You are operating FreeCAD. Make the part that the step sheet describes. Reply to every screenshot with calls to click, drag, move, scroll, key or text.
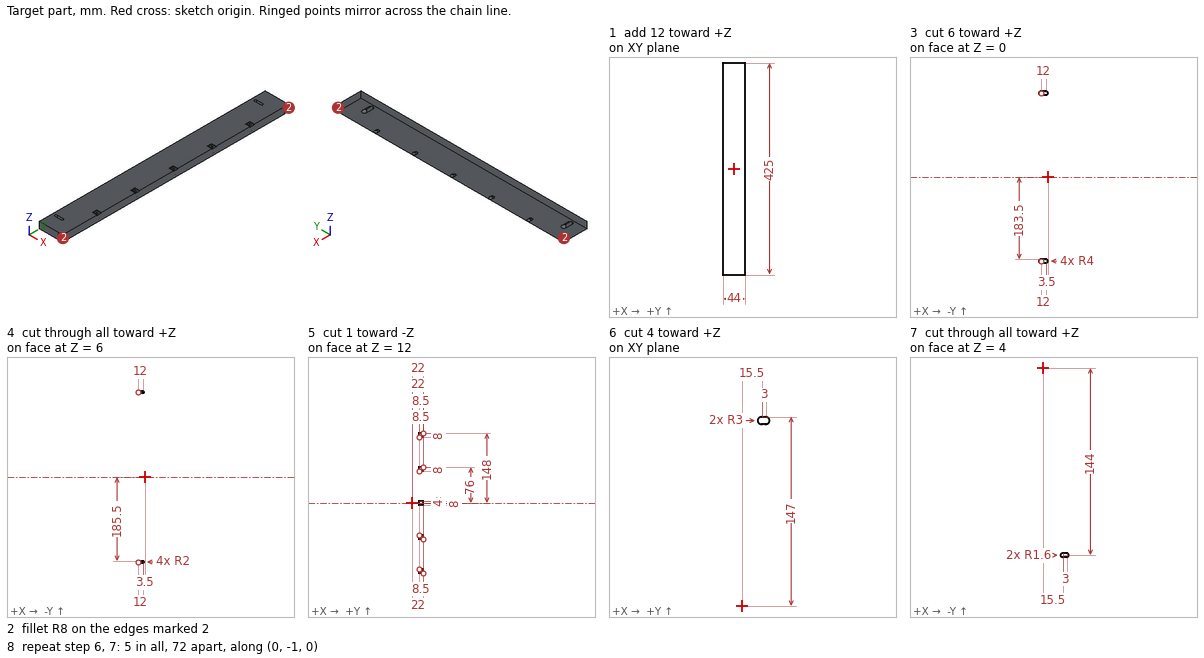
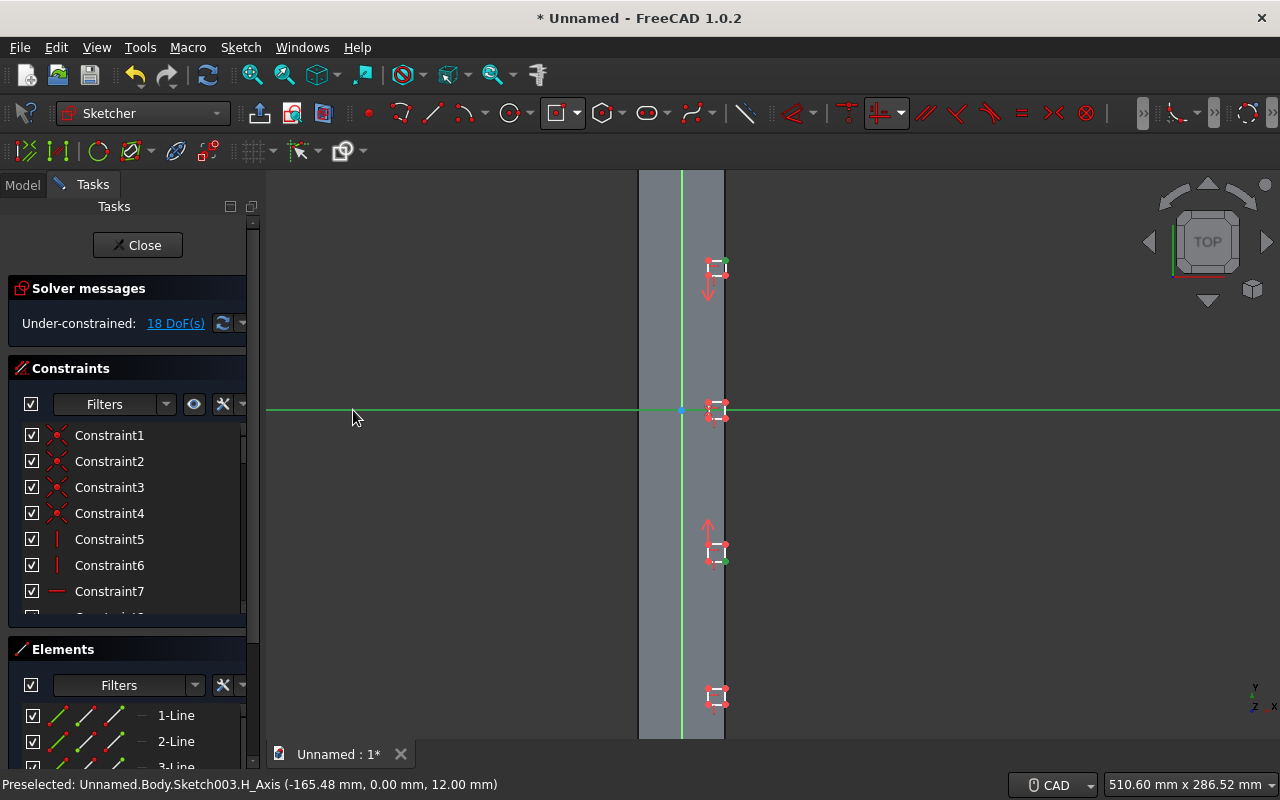
key(s)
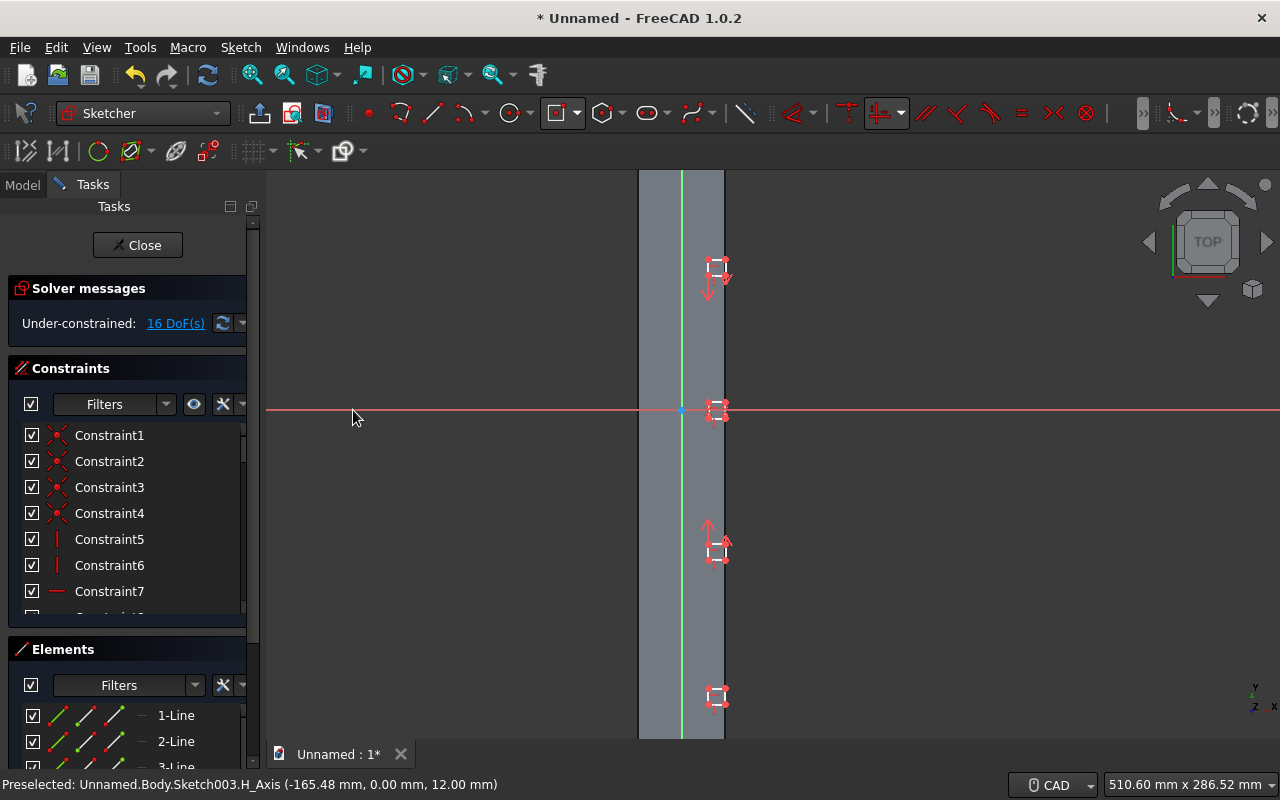
scroll(707, 545, down, 2)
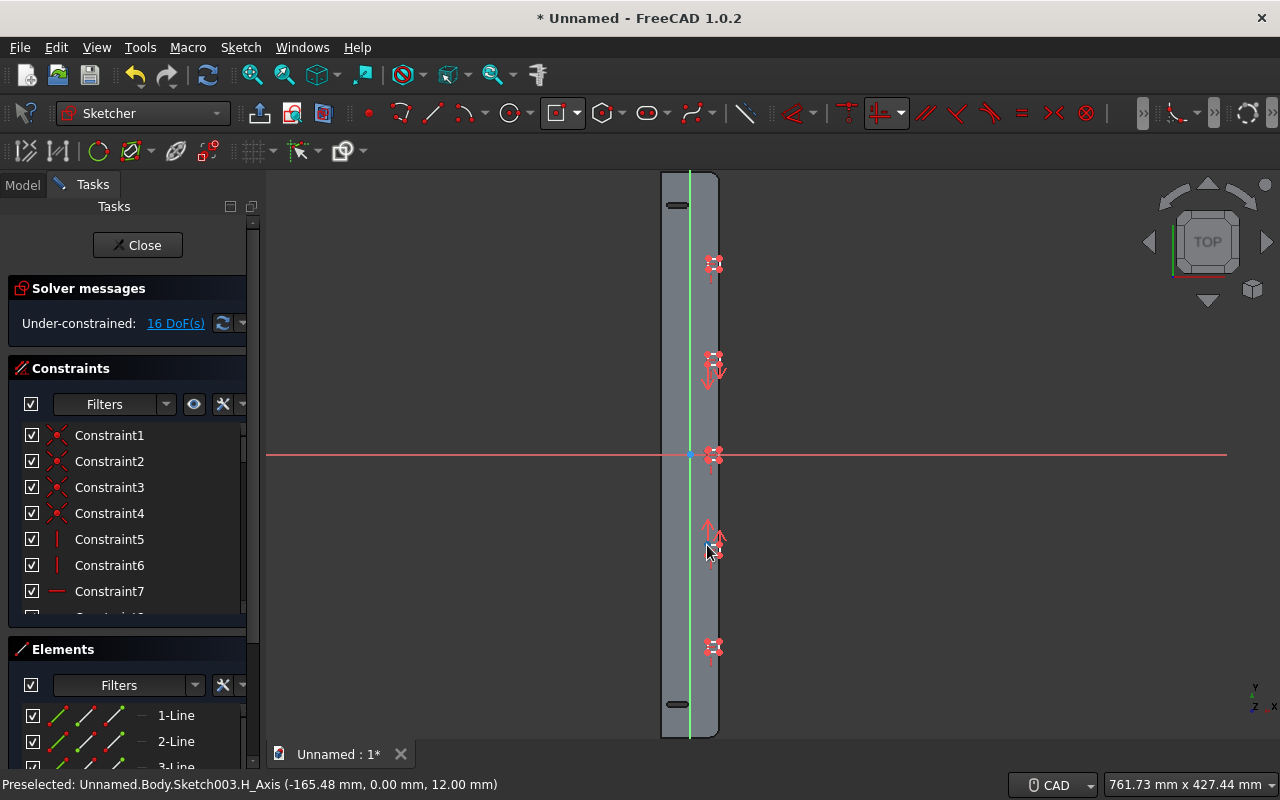
click(708, 269)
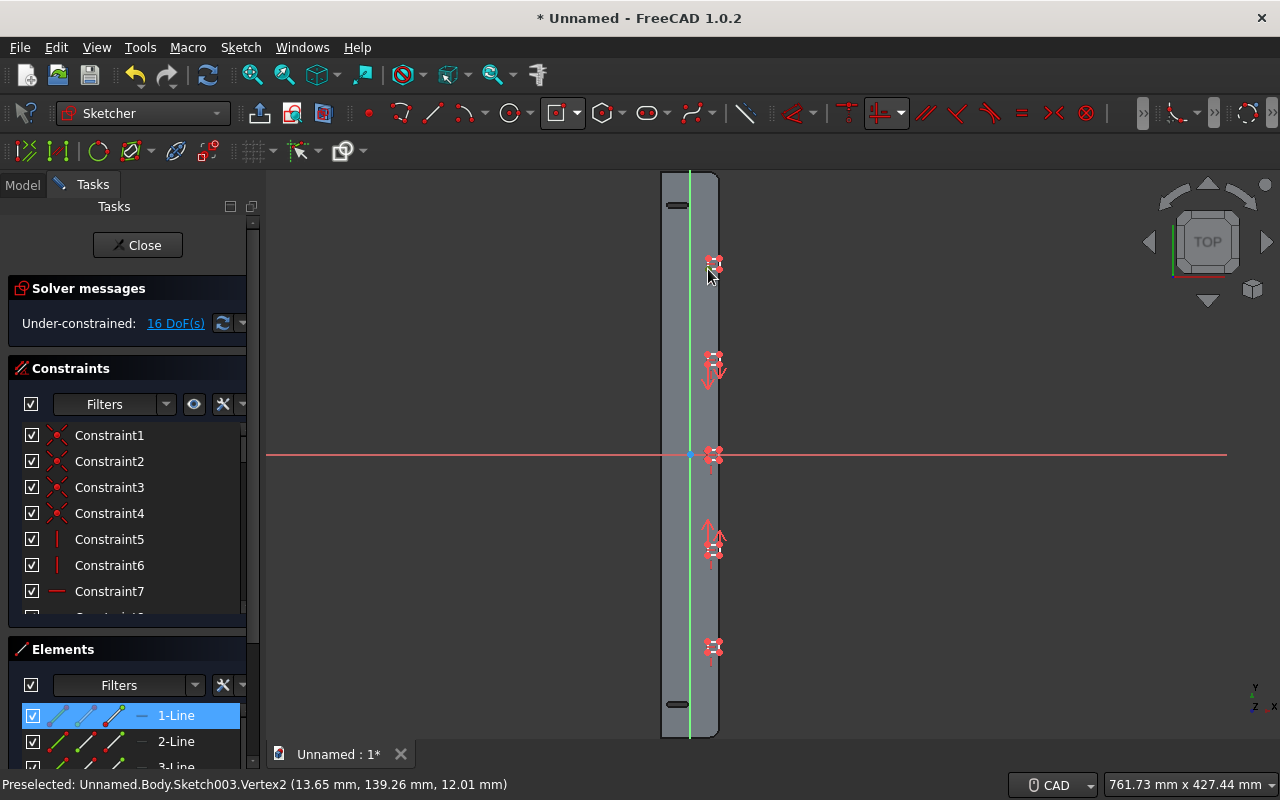
click(708, 642)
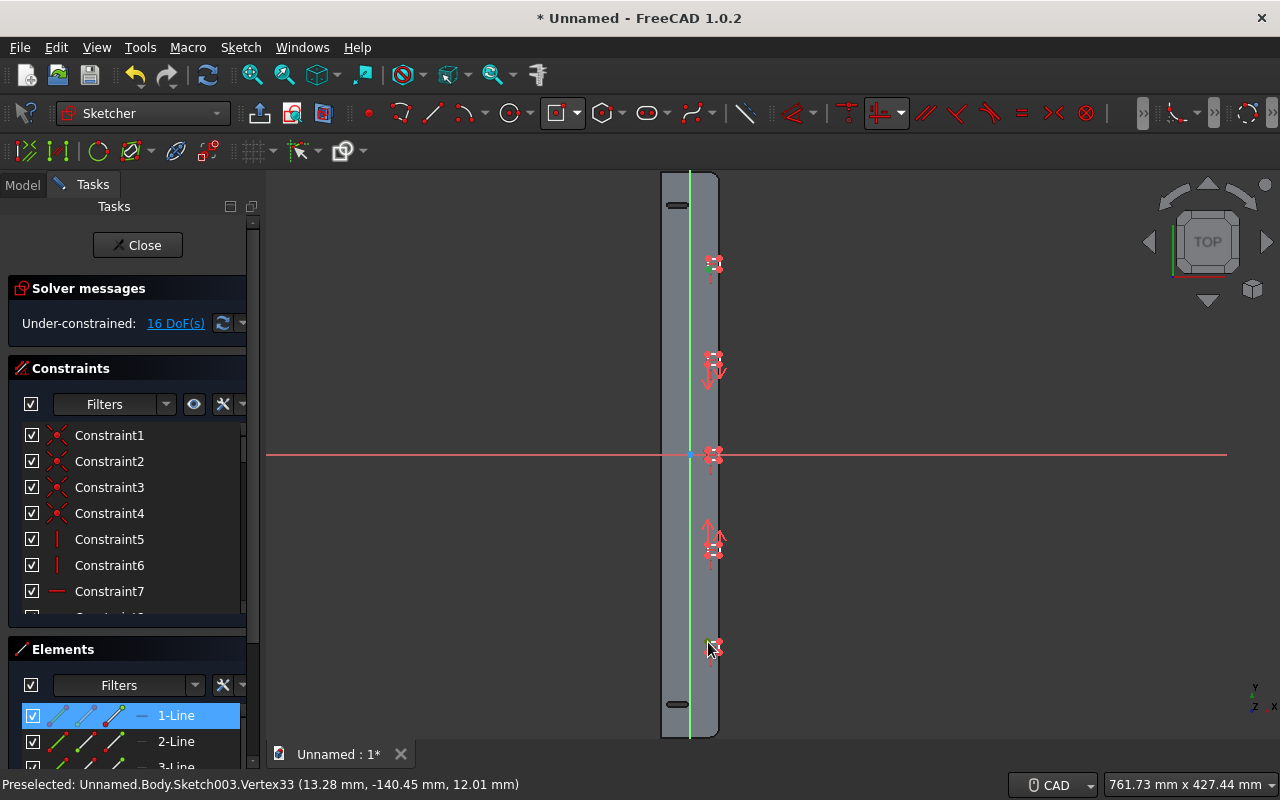
click(353, 455)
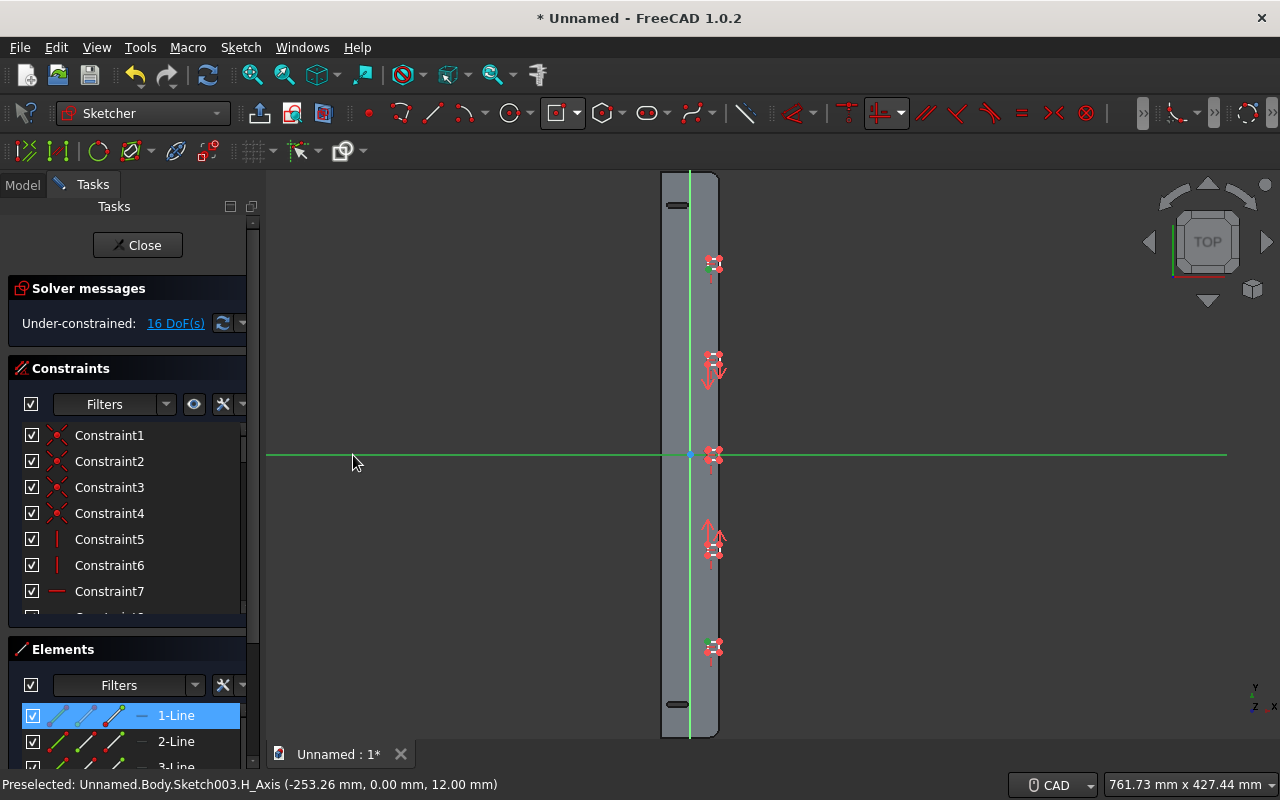
click(1054, 114)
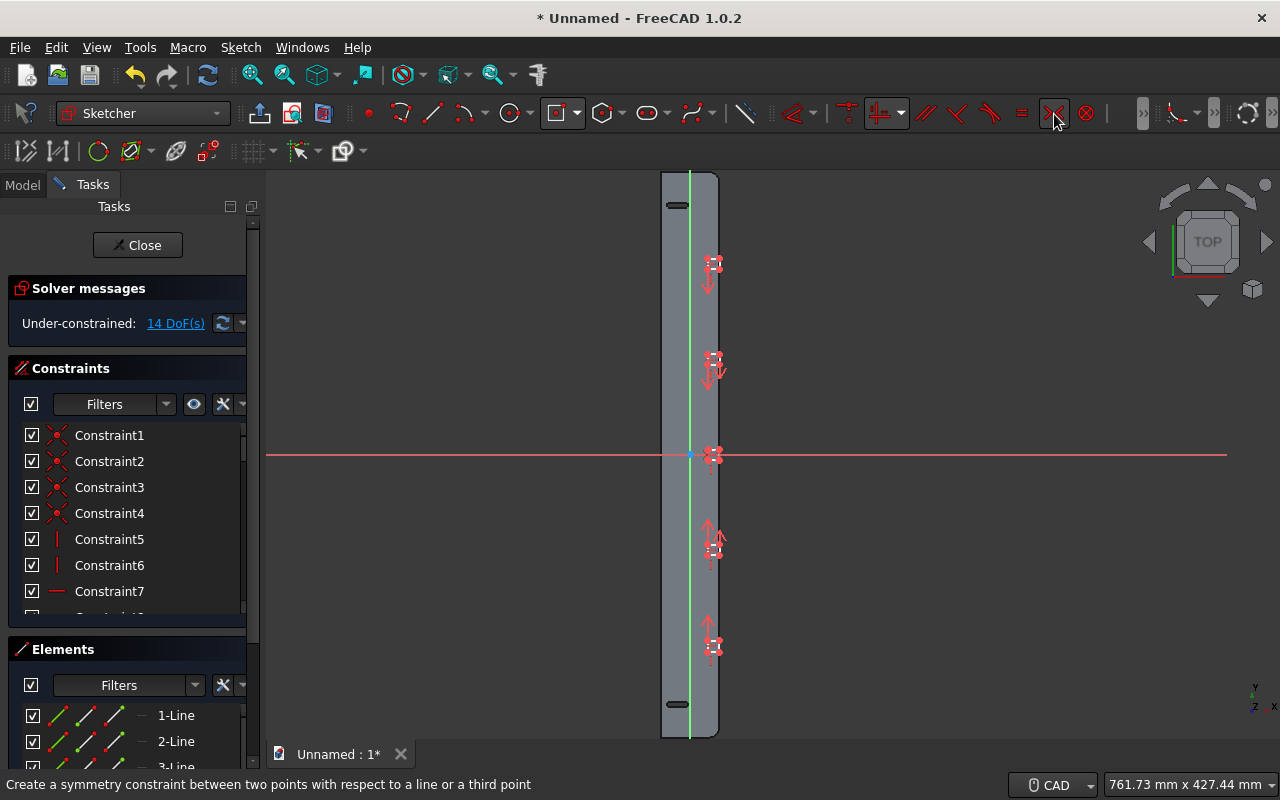
click(720, 259)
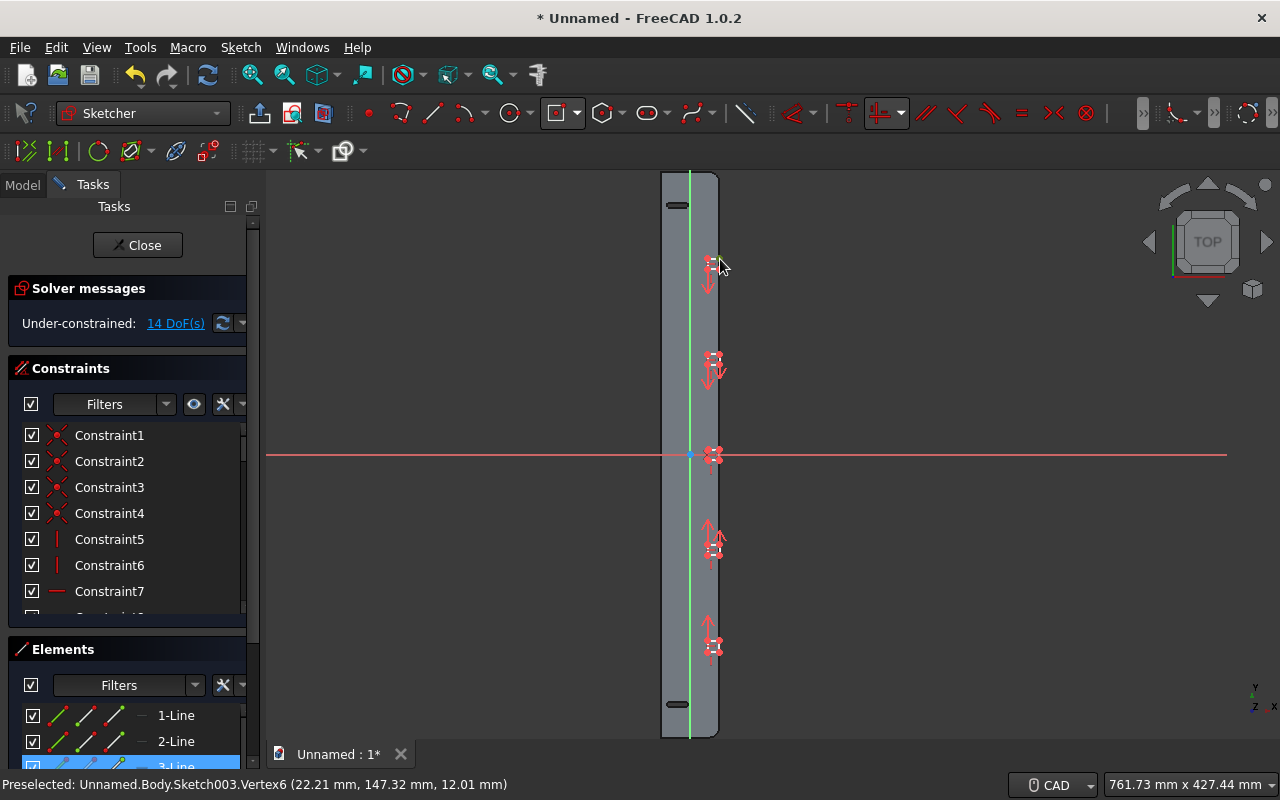
click(719, 652)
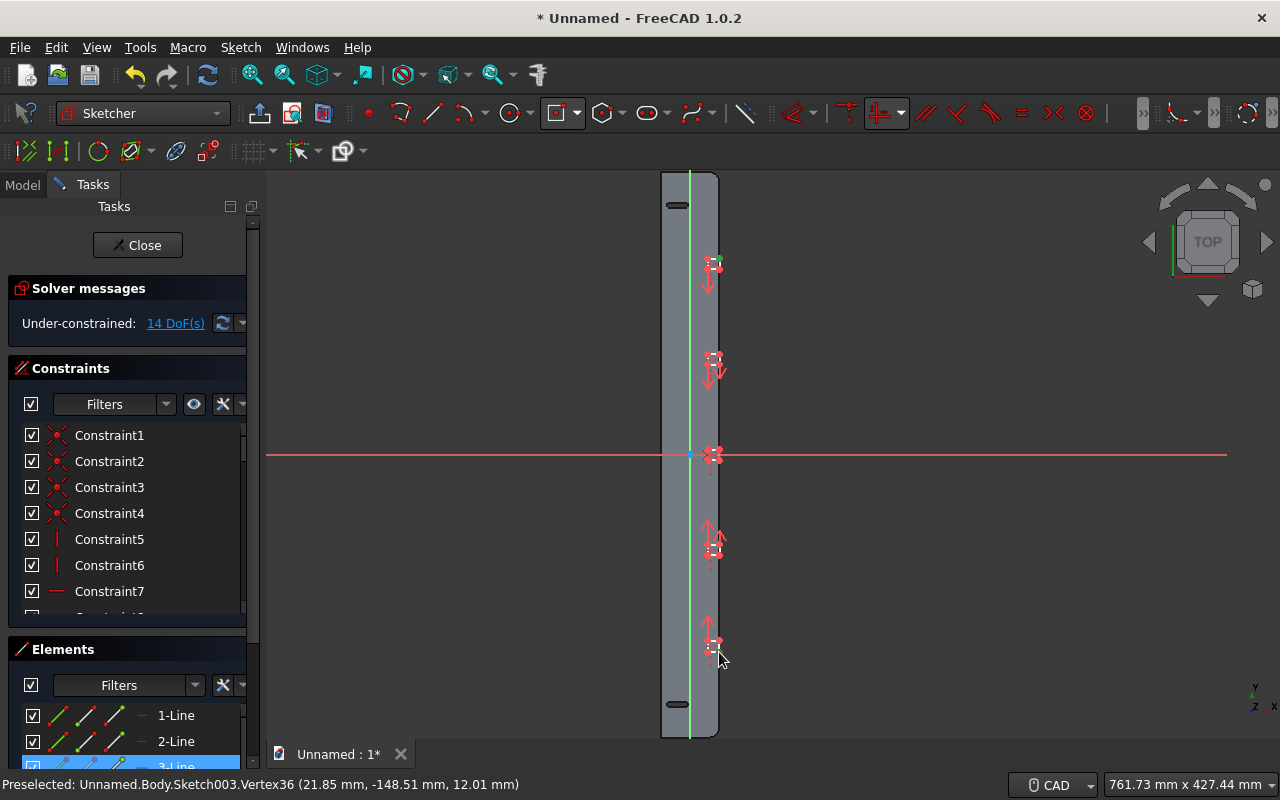
click(353, 455)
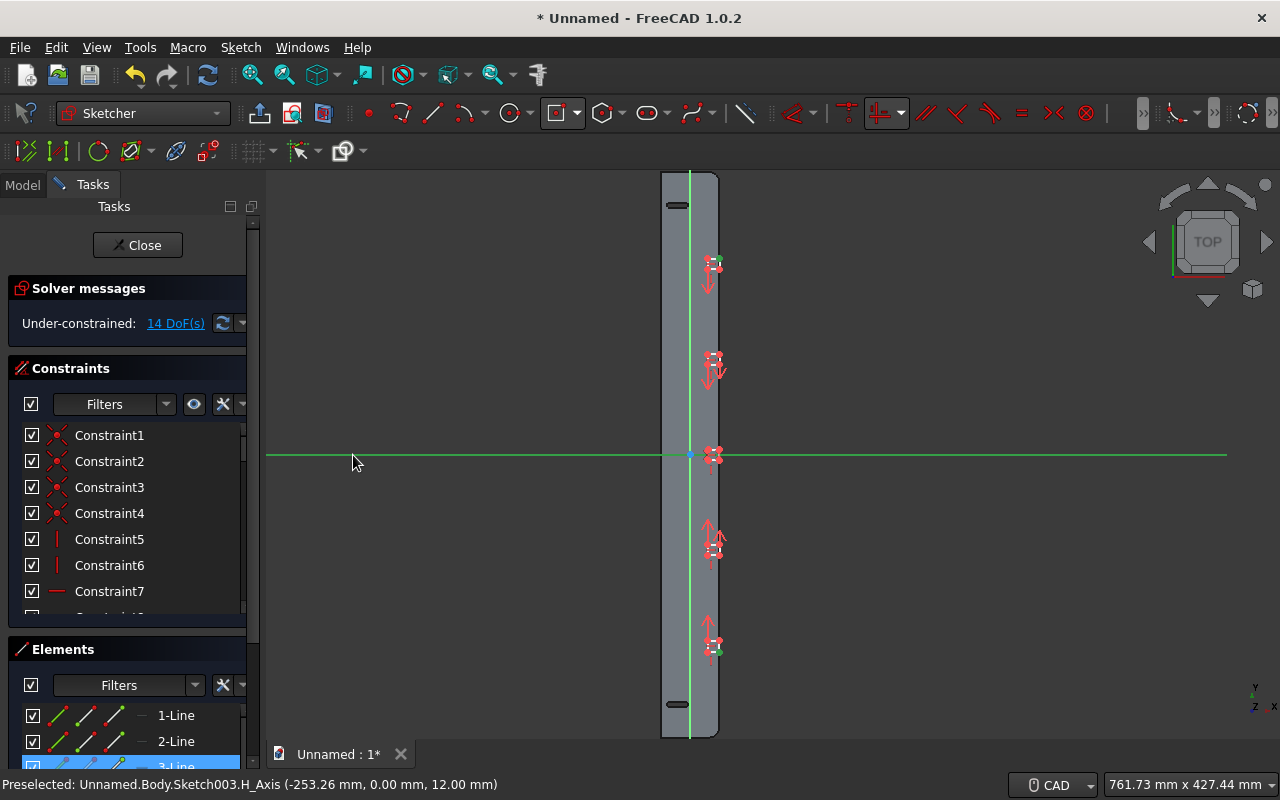
click(1054, 114)